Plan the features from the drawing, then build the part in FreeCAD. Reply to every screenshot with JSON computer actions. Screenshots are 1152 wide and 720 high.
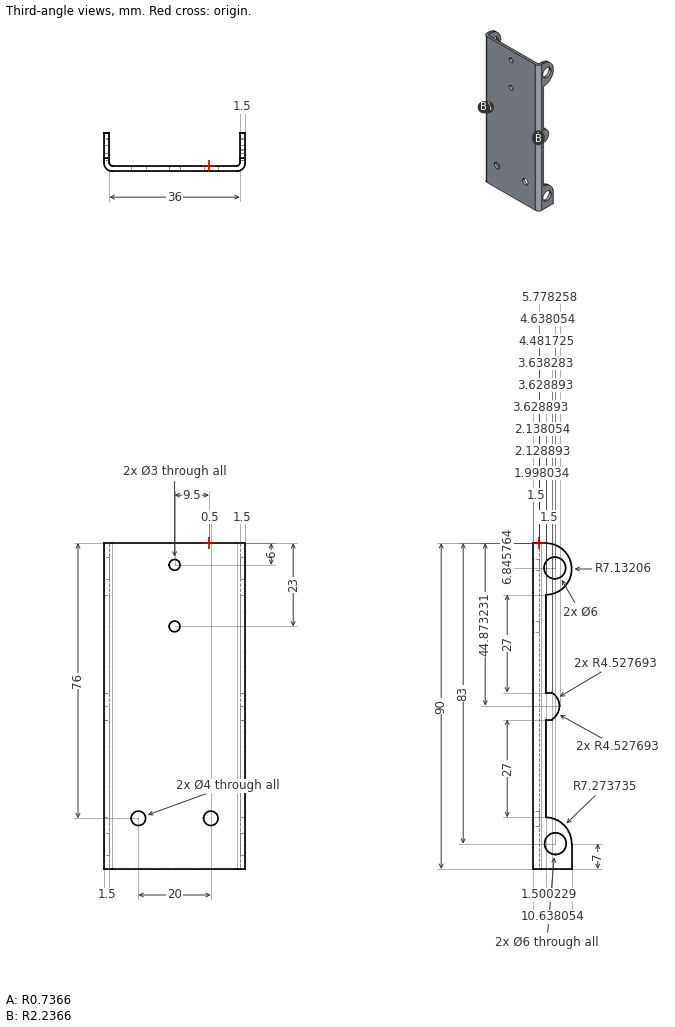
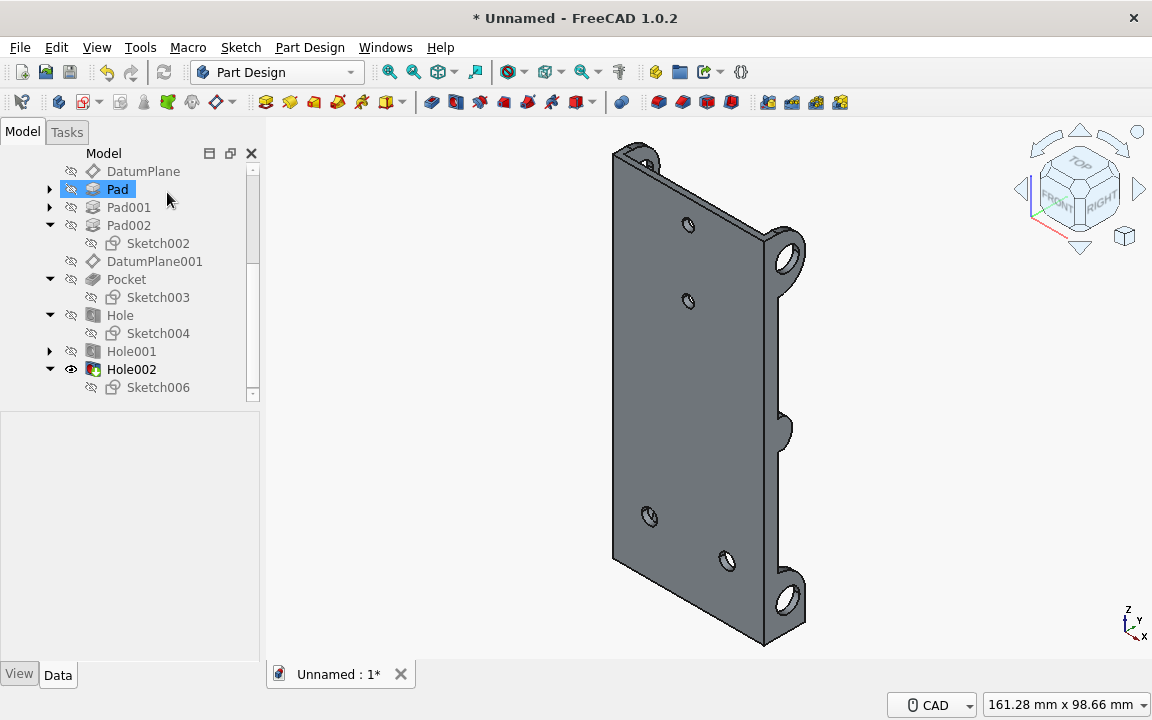
{"action": "key", "text": "2"}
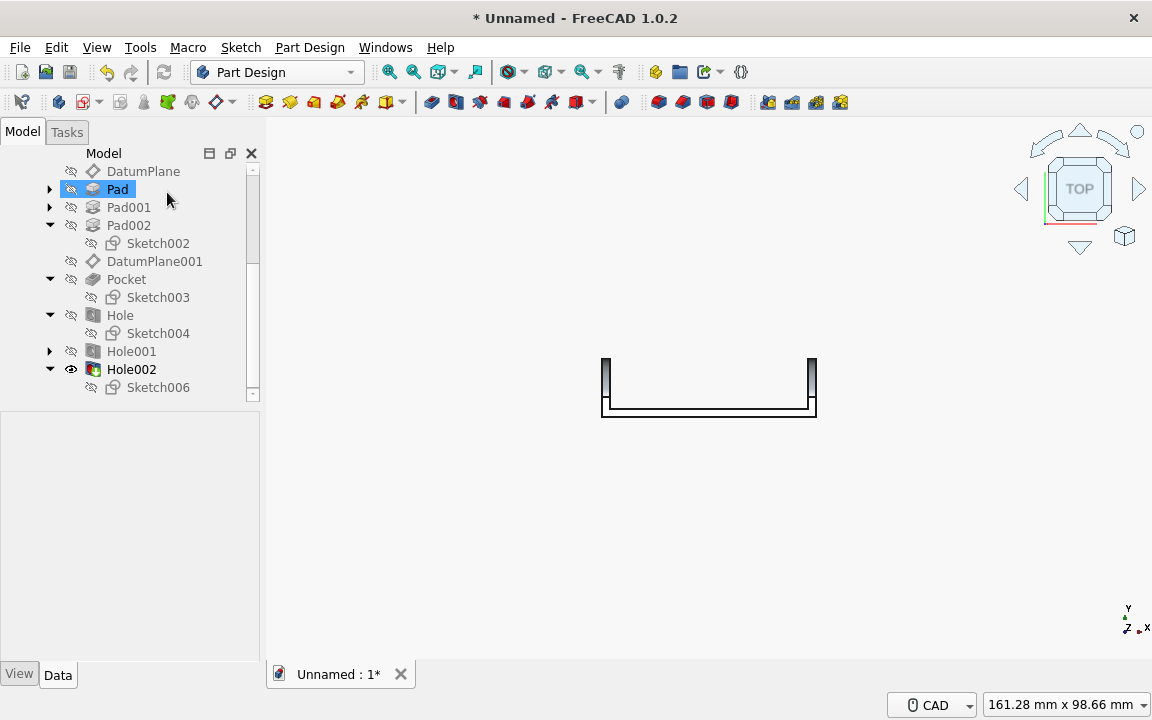
{"action": "left_click", "coordinate": [390, 72]}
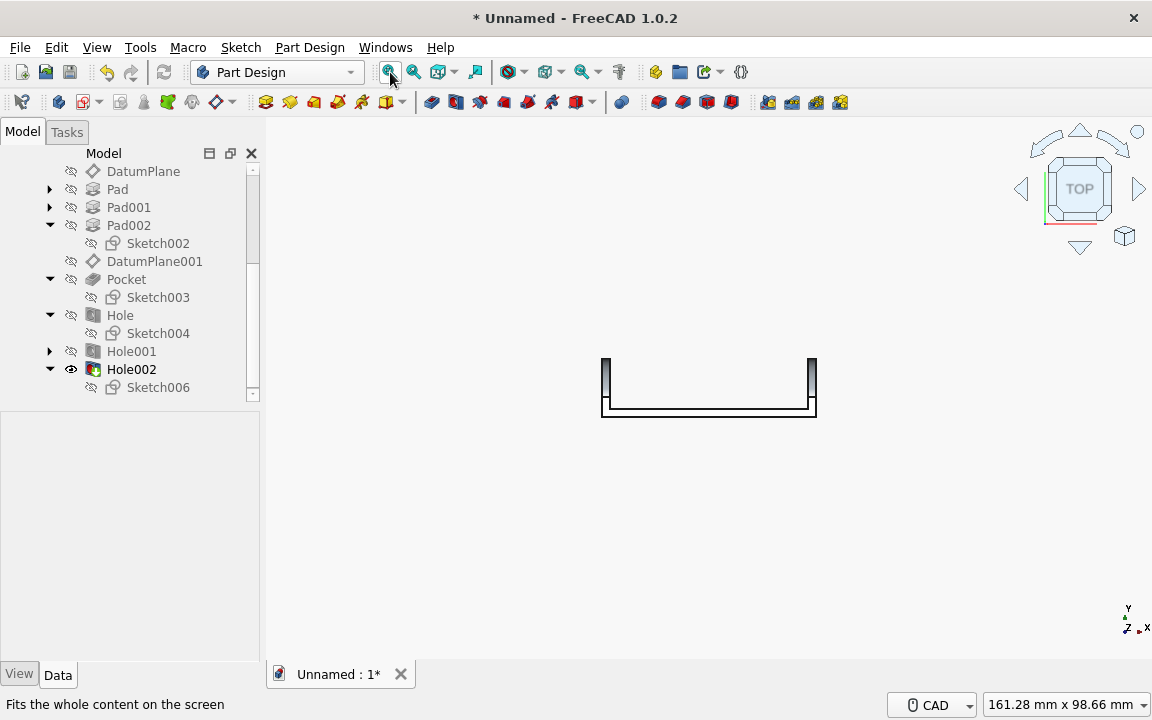
{"action": "key", "text": "1"}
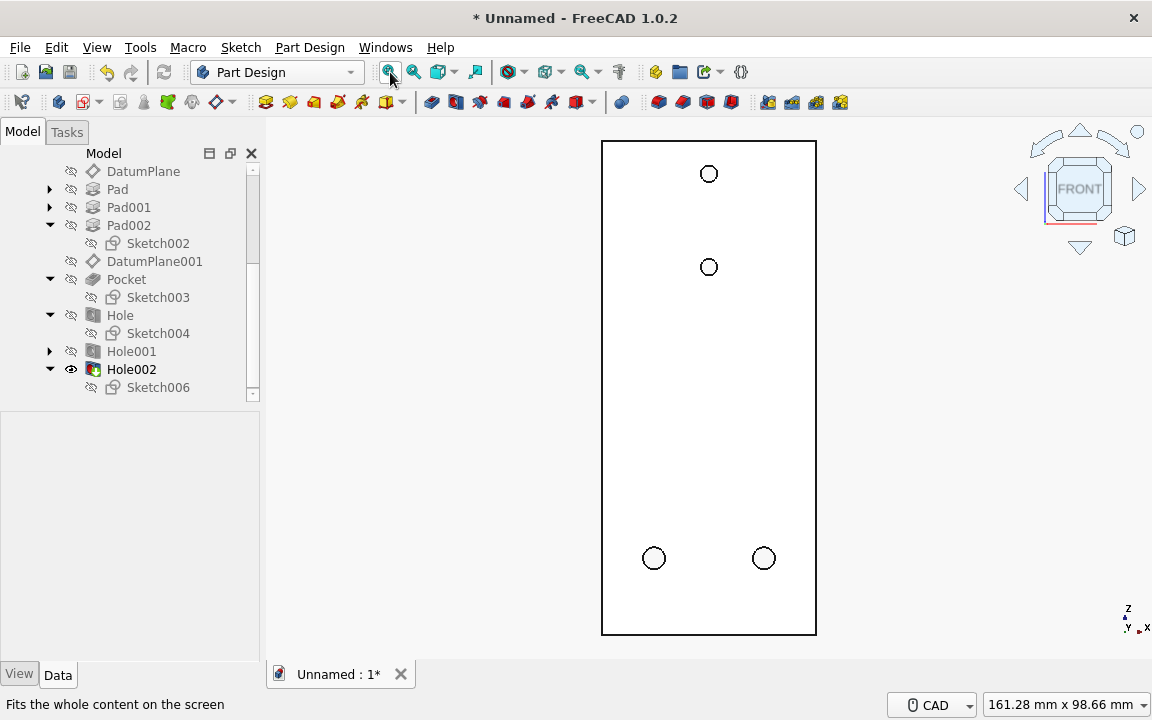
{"action": "key", "text": "3"}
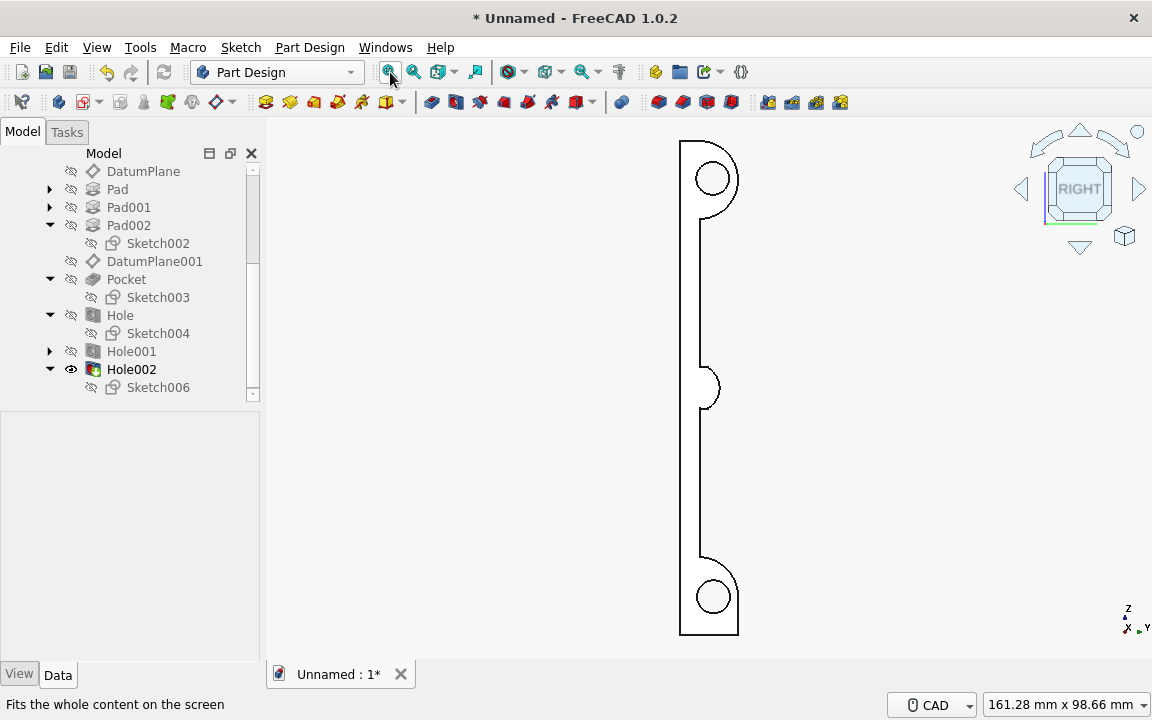
{"action": "key", "text": "5"}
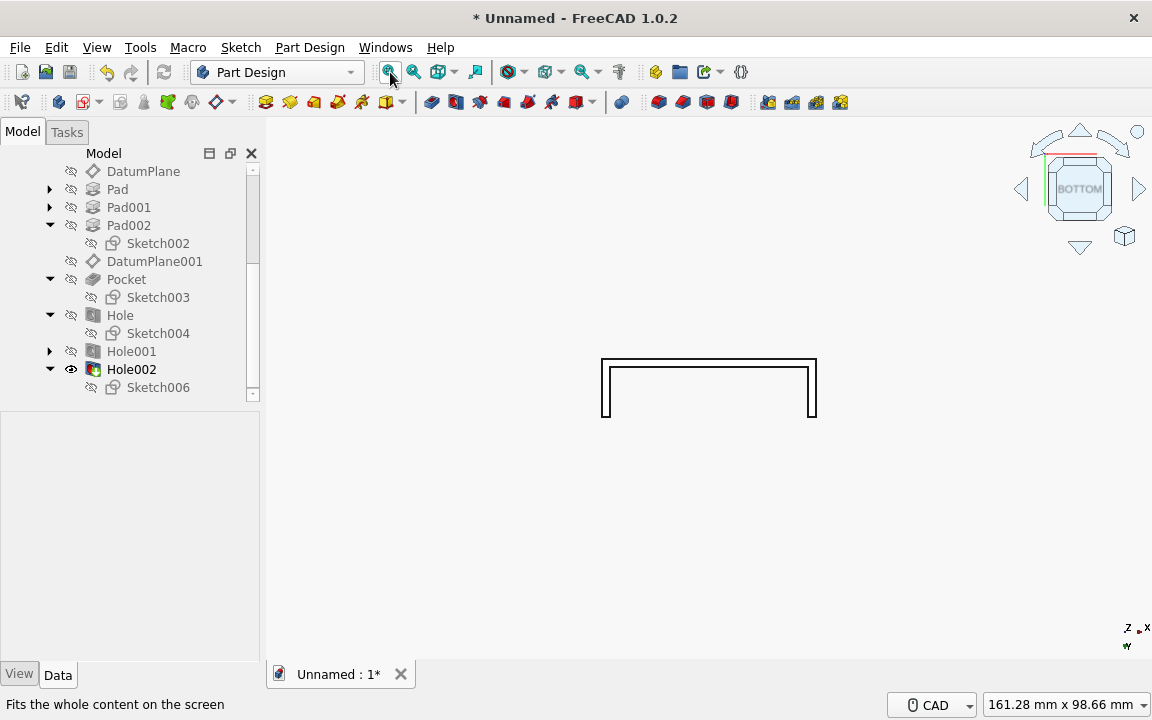
{"action": "left_click", "coordinate": [390, 72]}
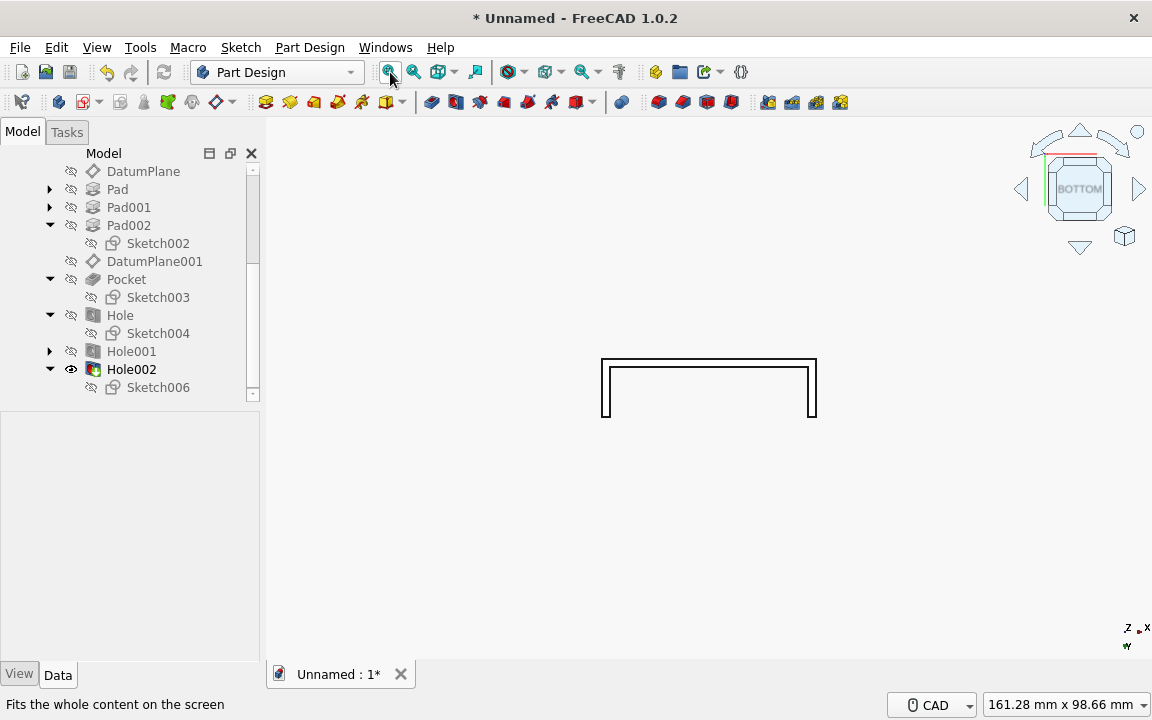
{"action": "key", "text": "4"}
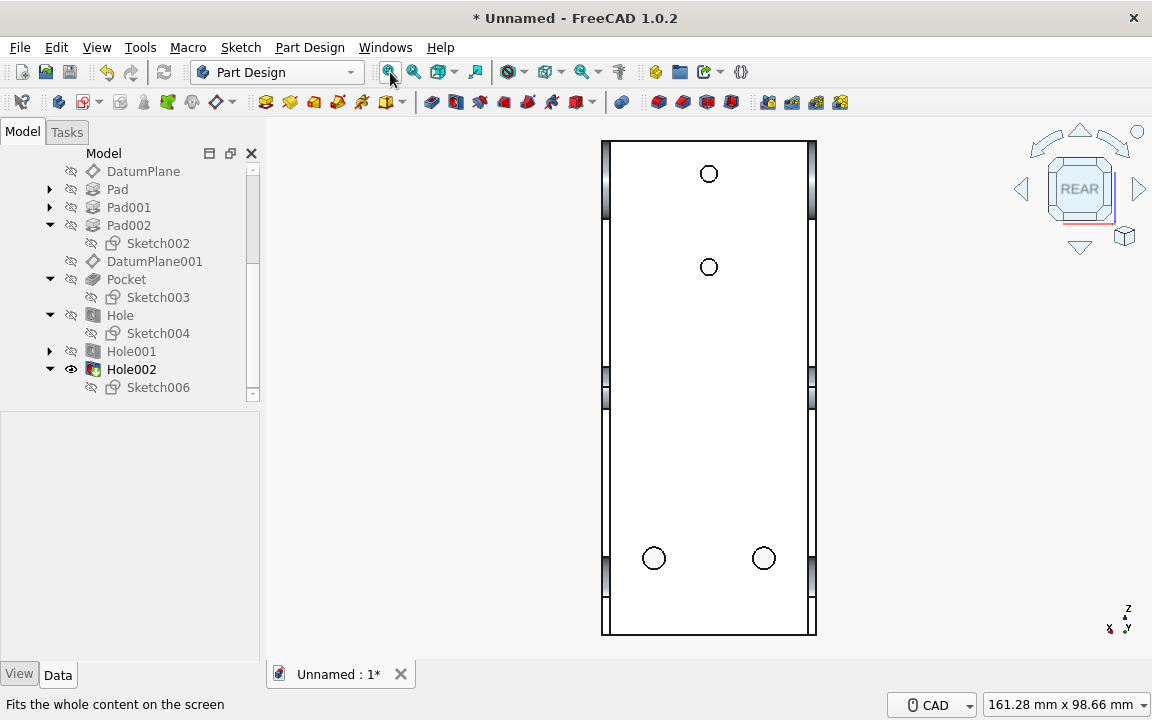
{"action": "key", "text": "6"}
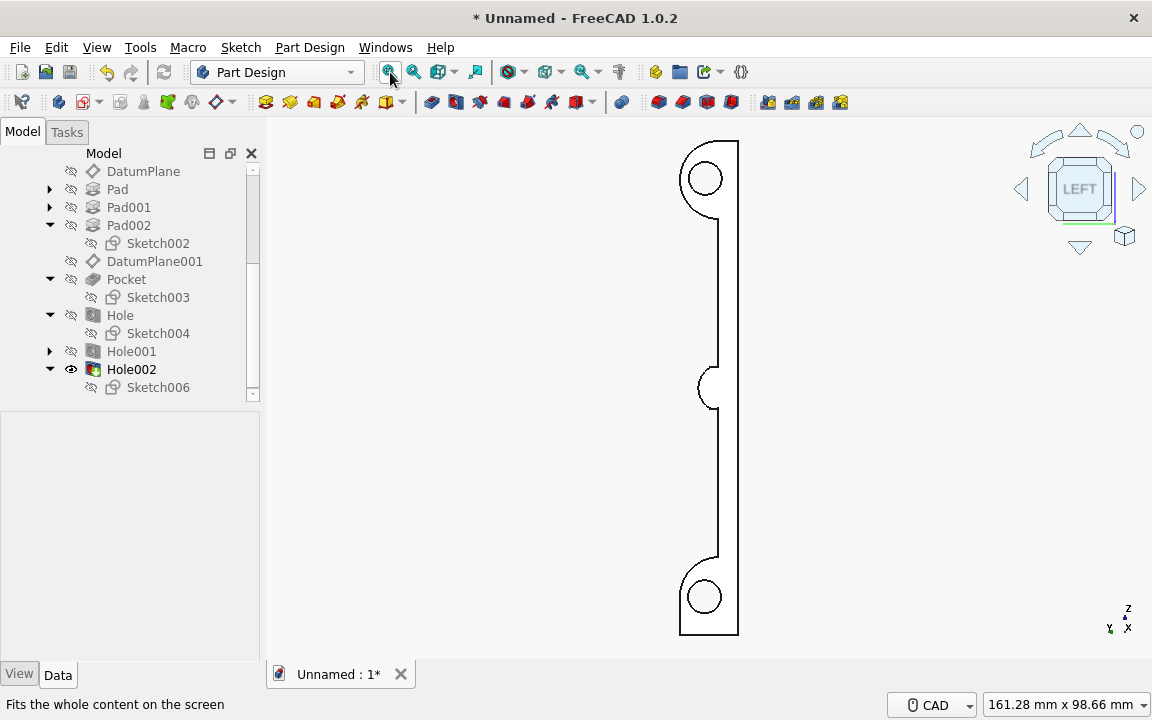
{"action": "key", "text": "v 3"}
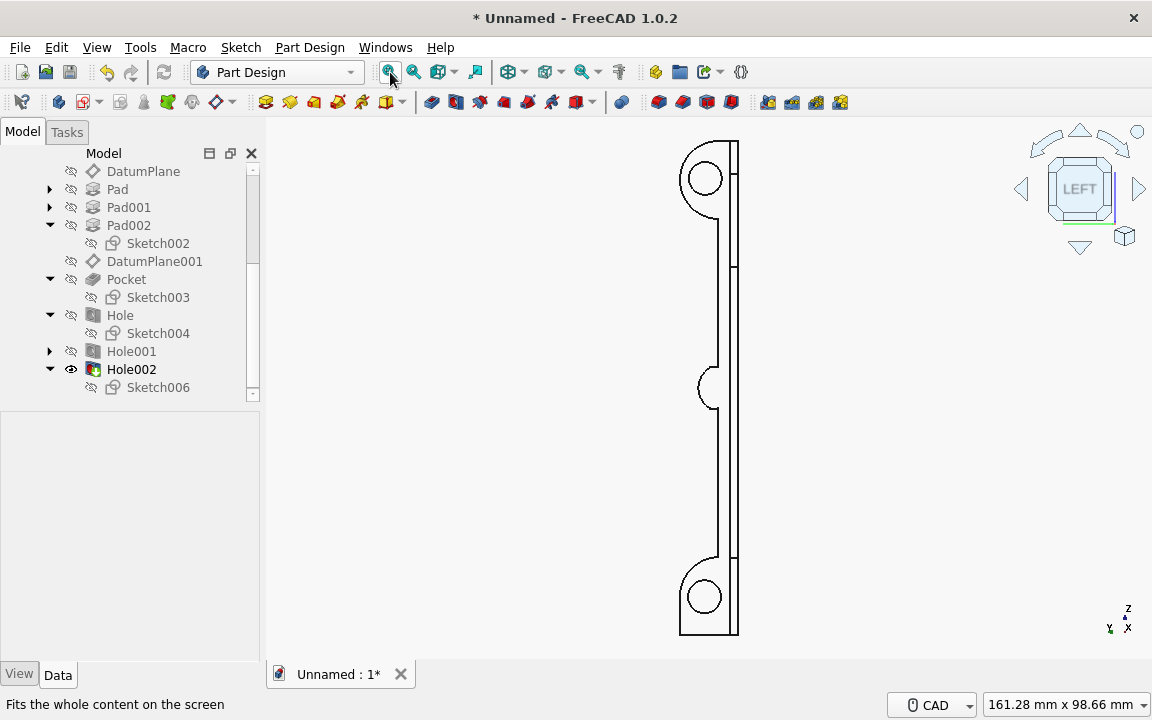
{"action": "key", "text": "0"}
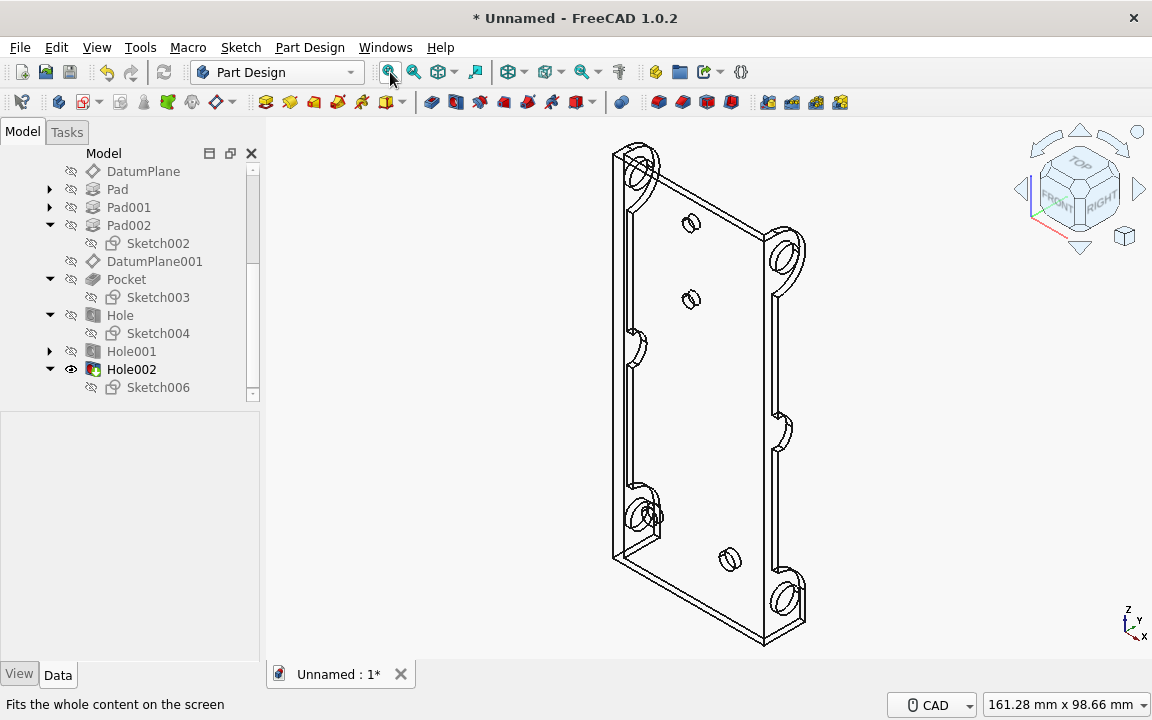
{"action": "left_click", "coordinate": [624, 355]}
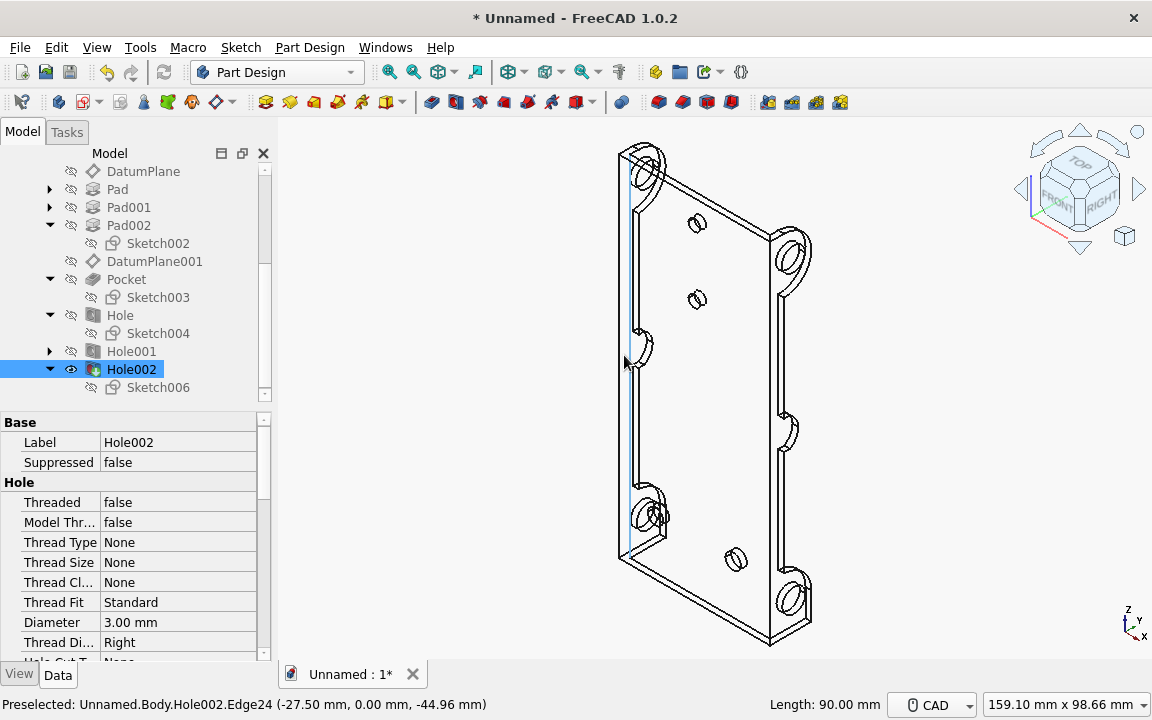
{"action": "scroll", "coordinate": [770, 436], "scroll_direction": "up", "scroll_amount": 6}